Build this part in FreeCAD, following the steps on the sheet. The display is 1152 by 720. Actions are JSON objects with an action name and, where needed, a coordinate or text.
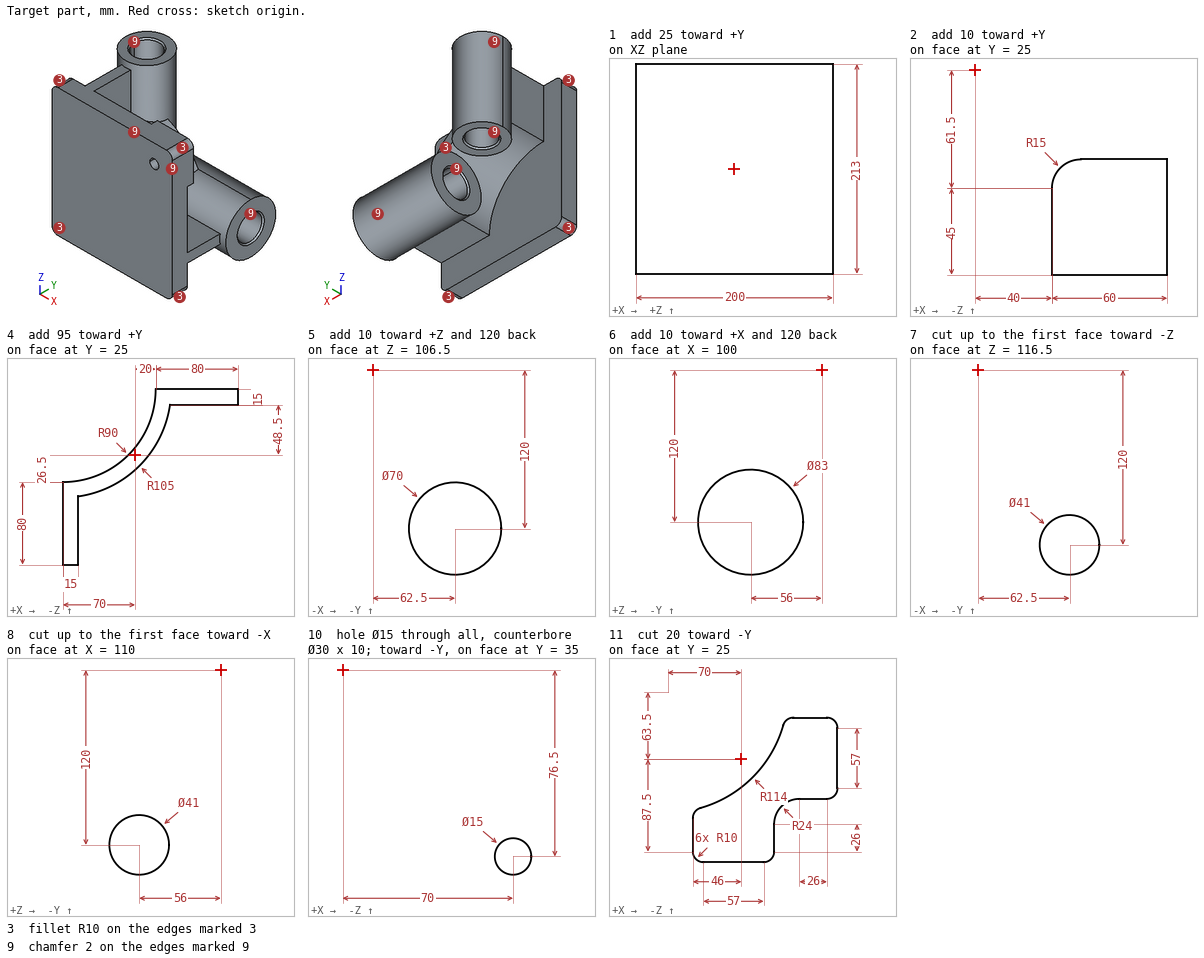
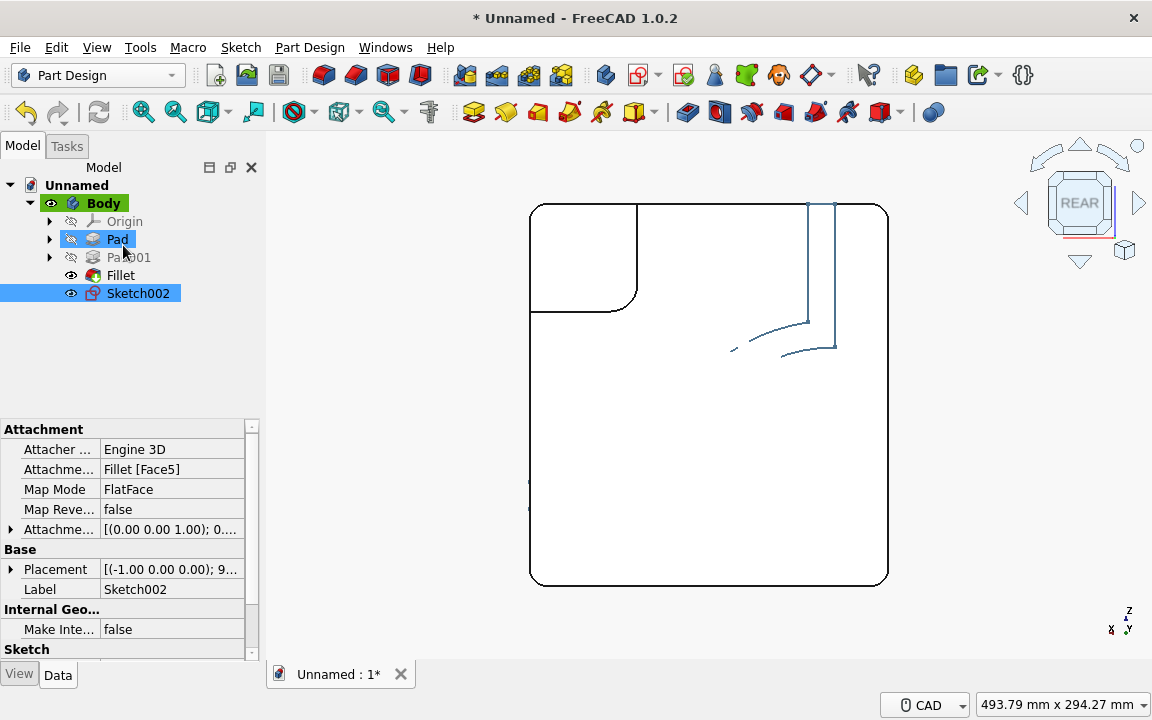
{"action": "left_click", "coordinate": [474, 112]}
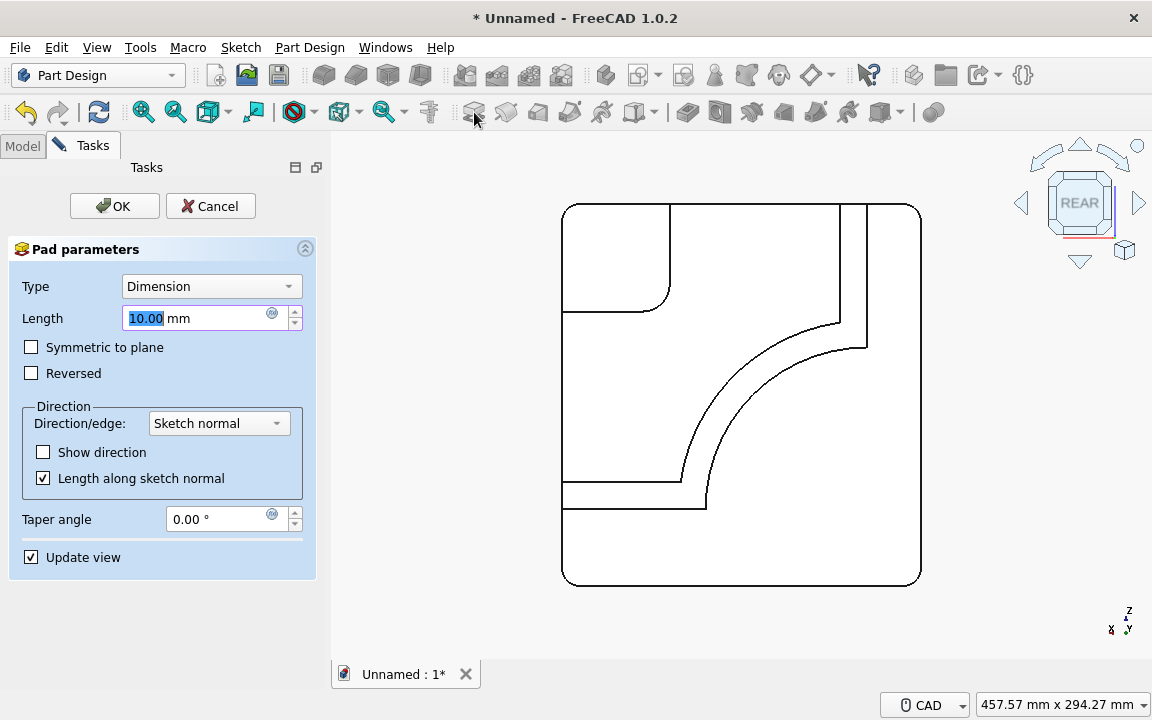
{"action": "type", "text": "95"}
{"action": "key", "text": "Tab"}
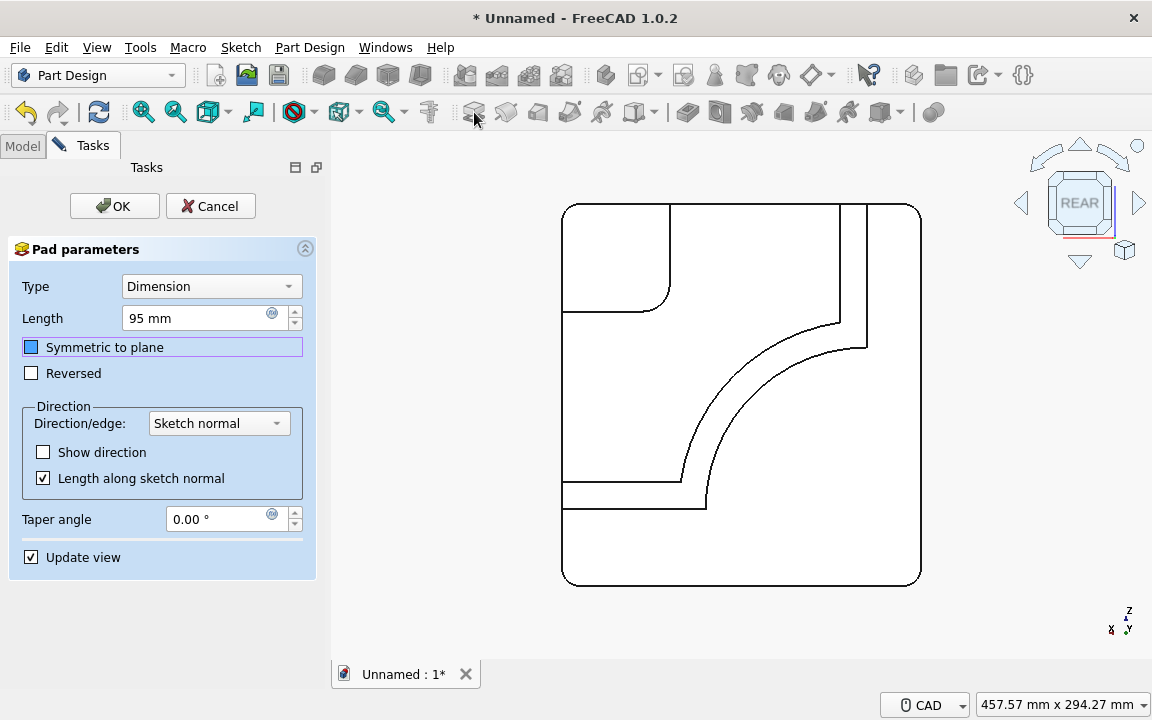
{"action": "left_click", "coordinate": [115, 206]}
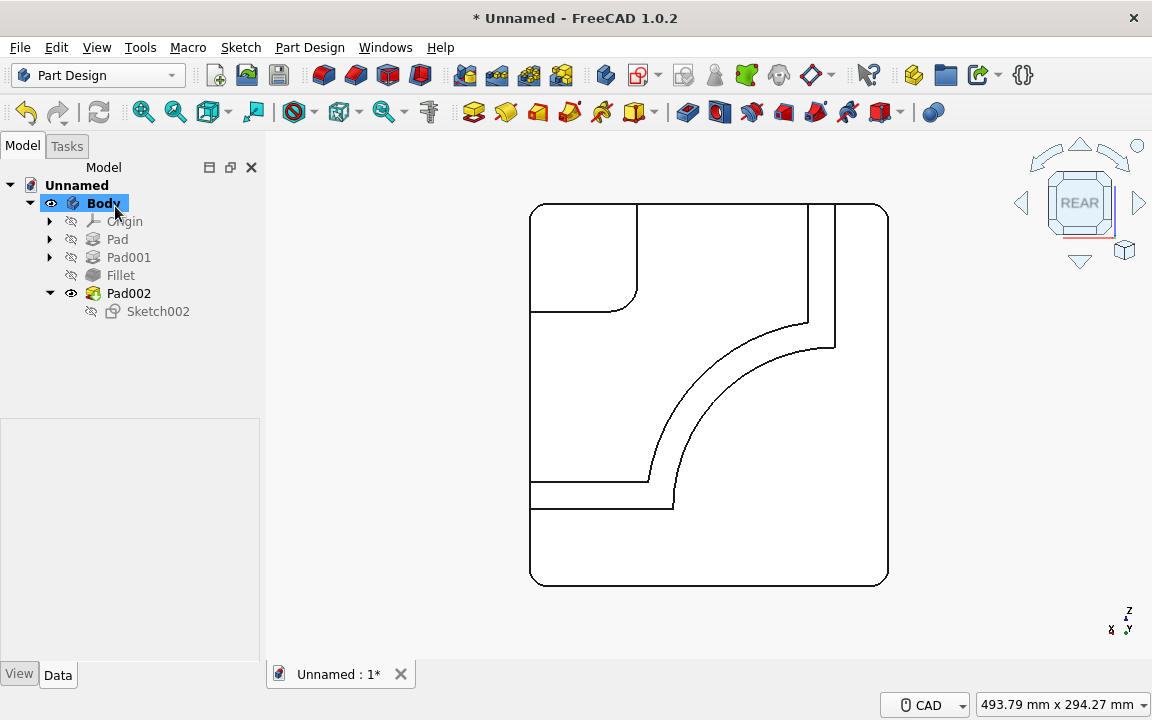
{"action": "key", "text": "0"}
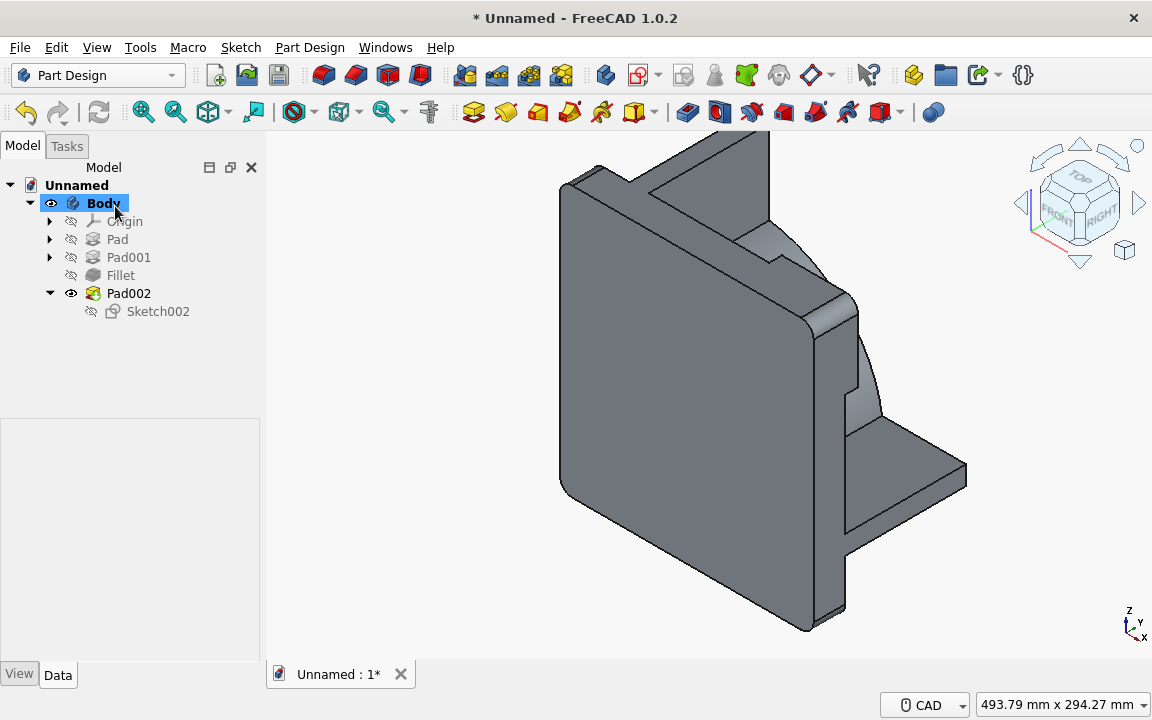
{"action": "left_click", "coordinate": [144, 112]}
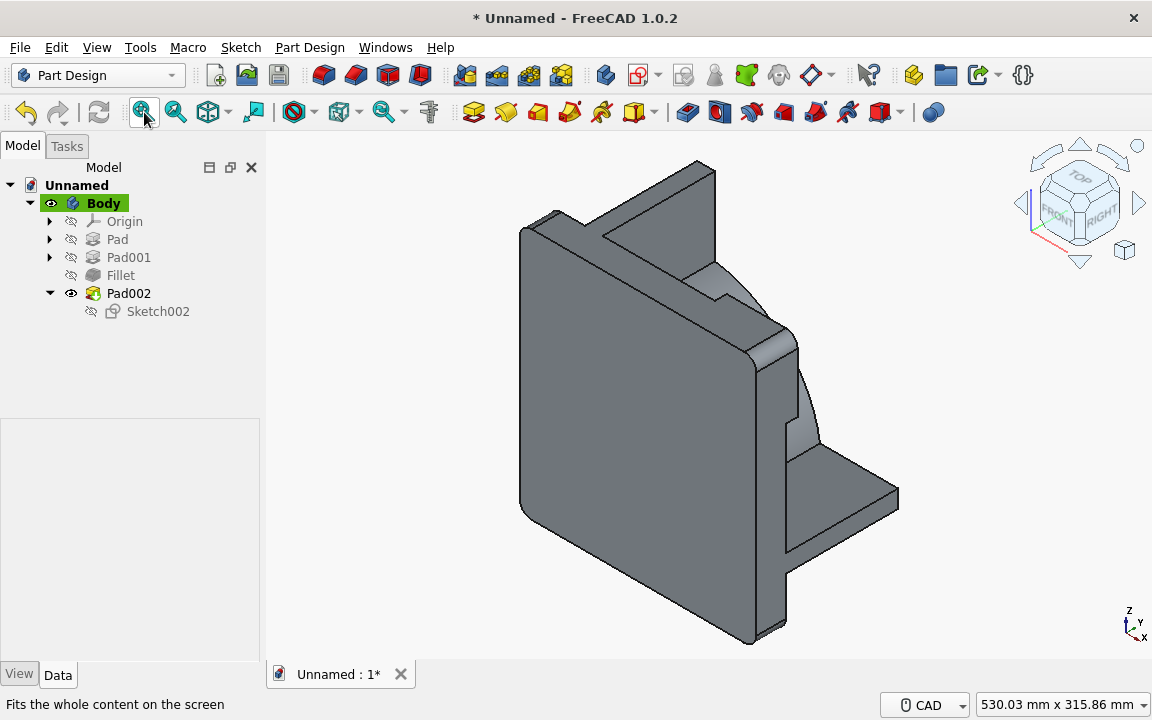
{"action": "left_click", "coordinate": [760, 325]}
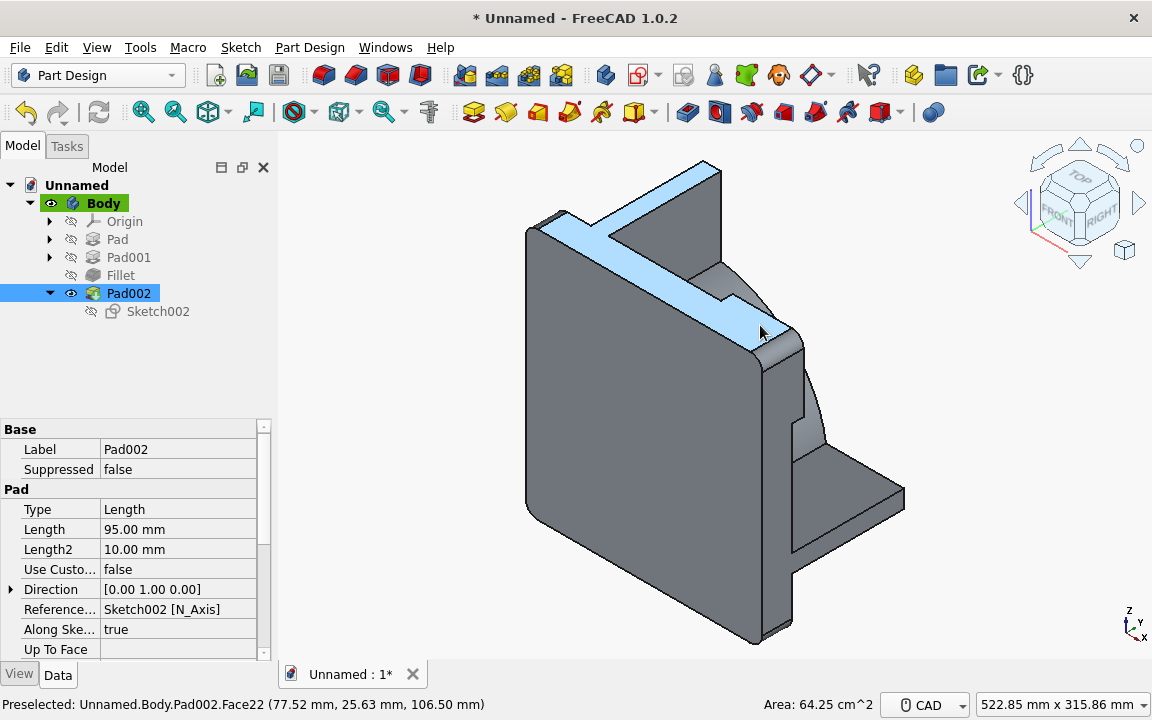
{"action": "left_click", "coordinate": [638, 76]}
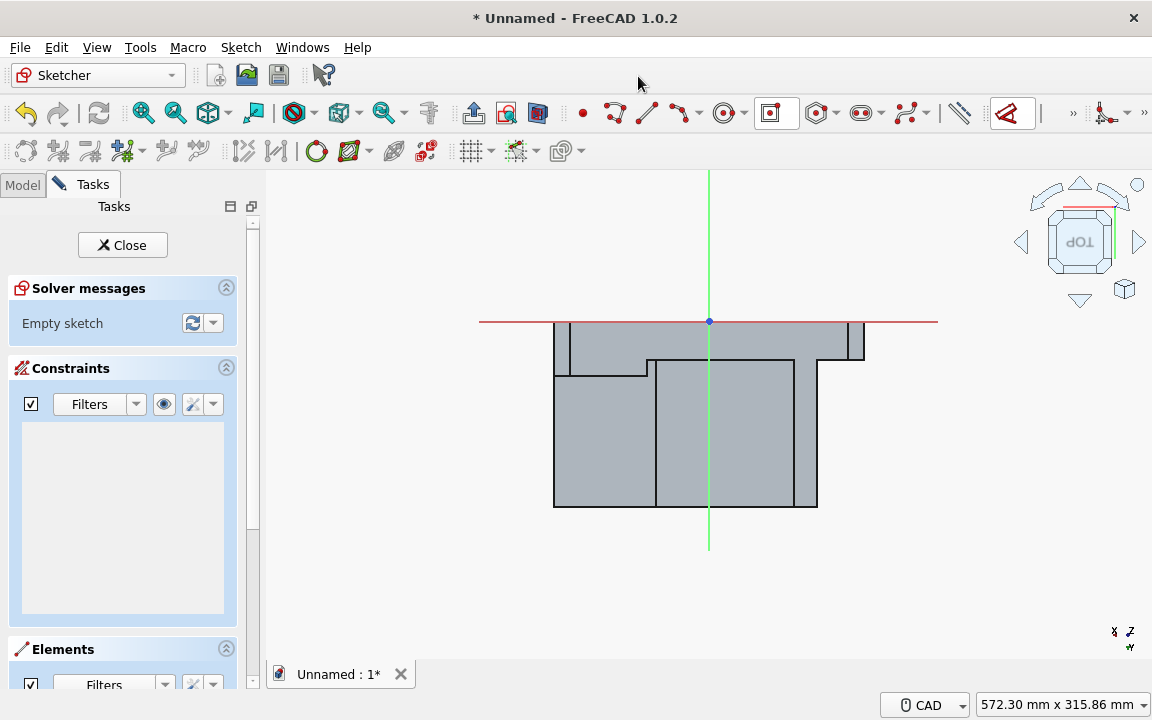
{"action": "left_click", "coordinate": [724, 114]}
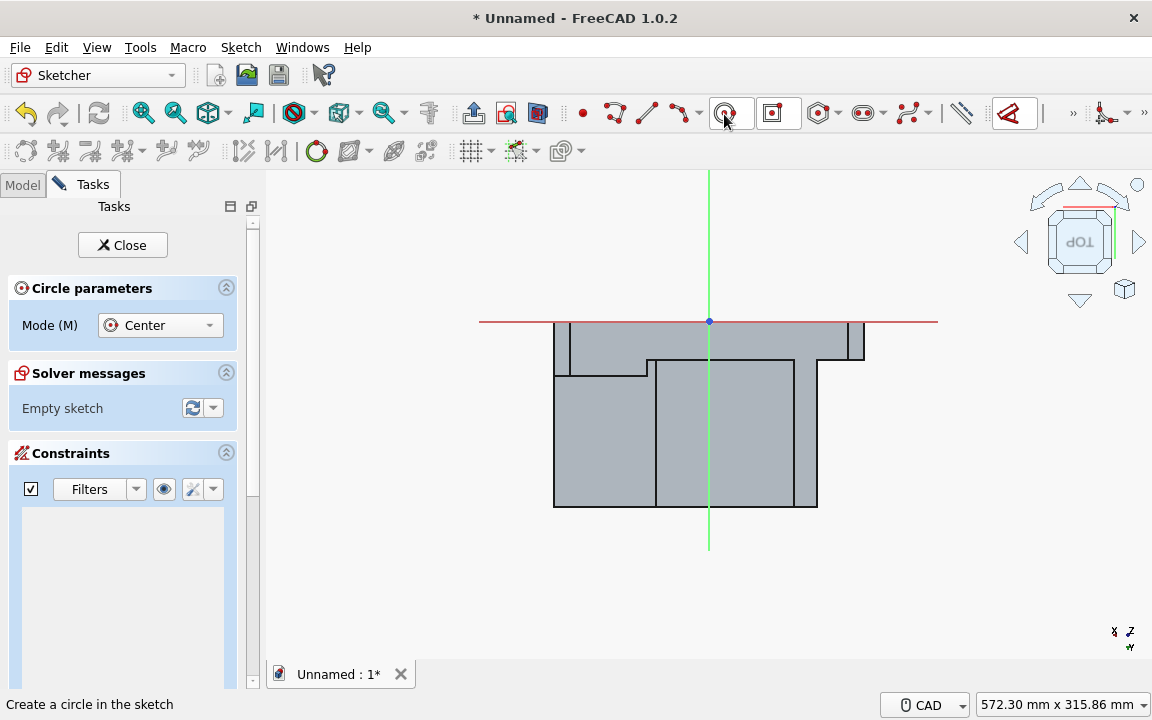
{"action": "left_click", "coordinate": [806, 507]}
{"action": "mouse_move", "coordinate": [844, 469]}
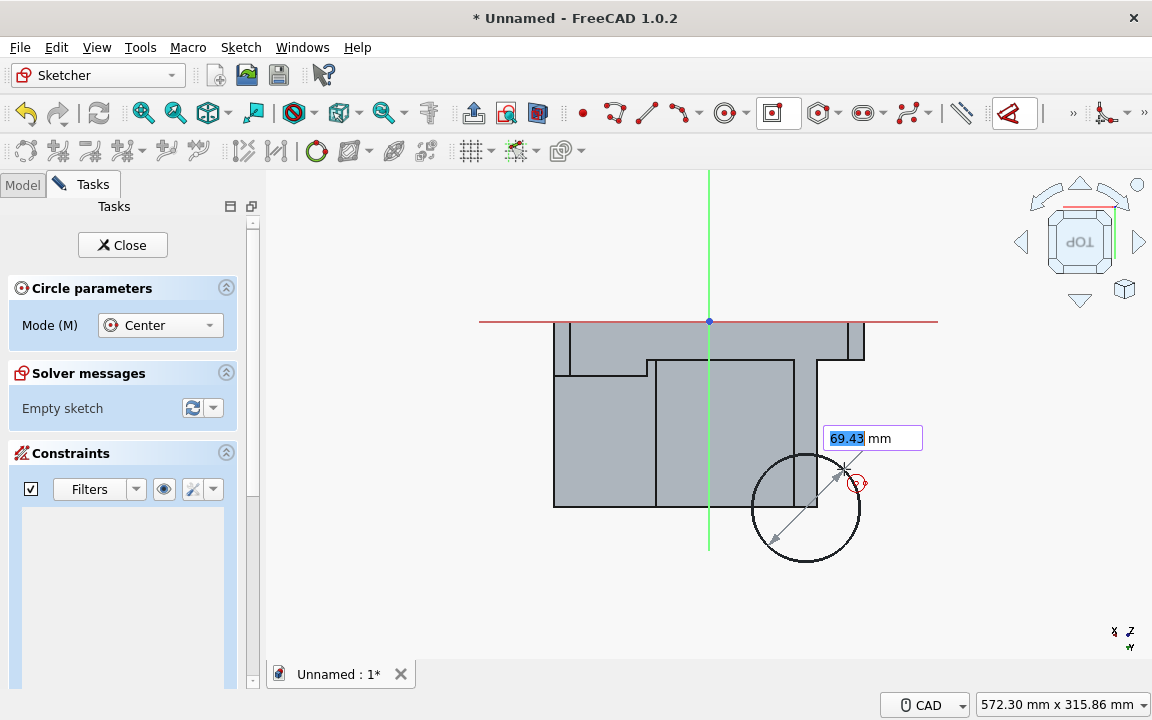
{"action": "type", "text": "70"}
{"action": "key", "text": "Return"}
{"action": "key", "text": "Escape"}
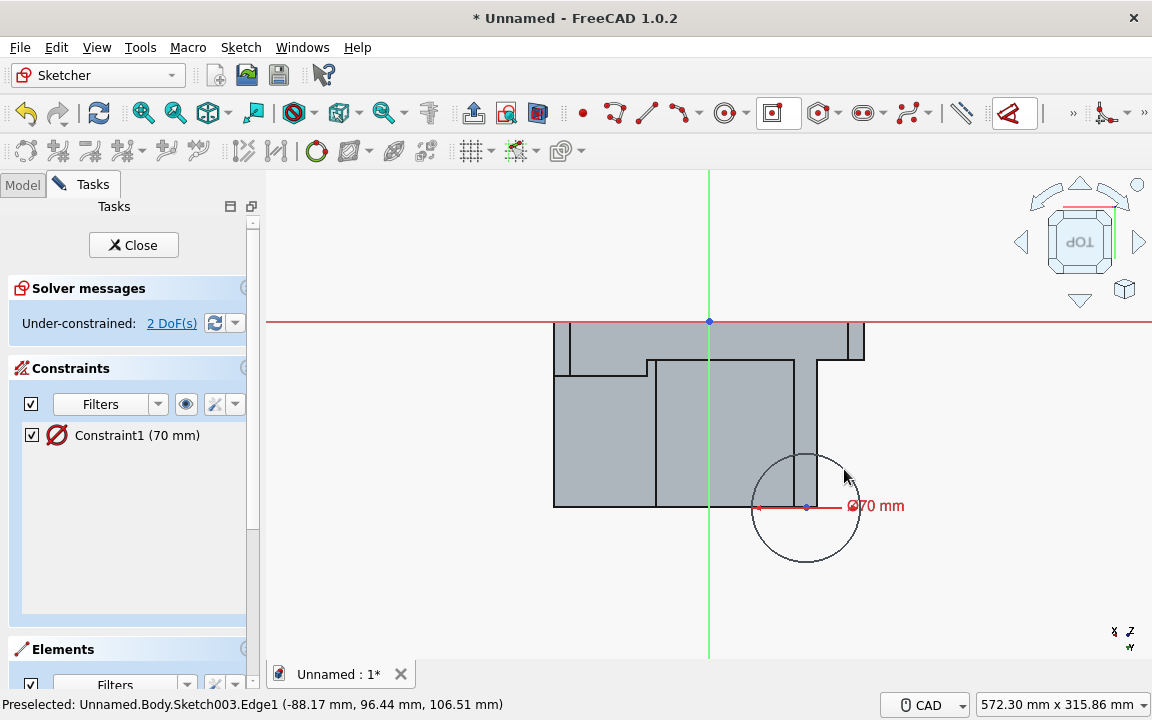
{"action": "left_click", "coordinate": [806, 508]}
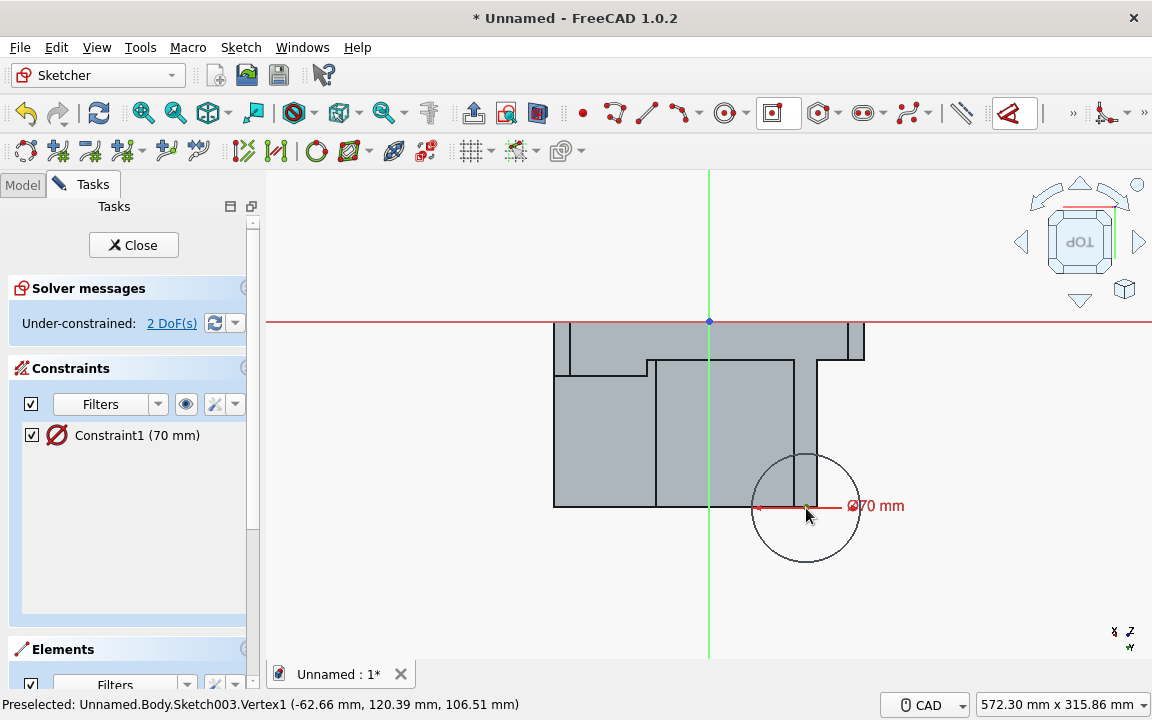
{"action": "left_click", "coordinate": [1032, 114]}